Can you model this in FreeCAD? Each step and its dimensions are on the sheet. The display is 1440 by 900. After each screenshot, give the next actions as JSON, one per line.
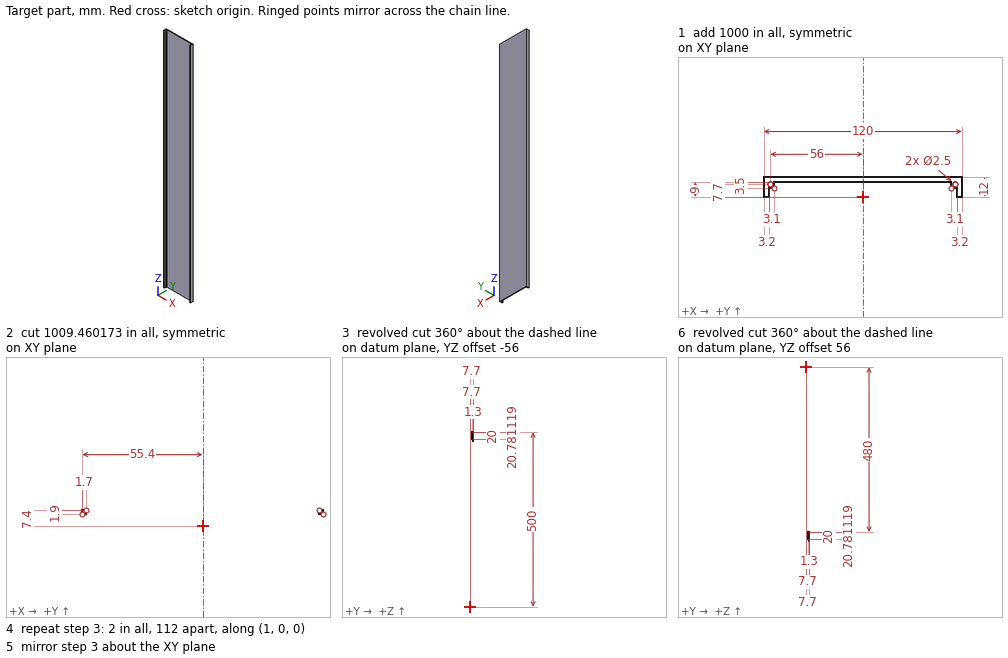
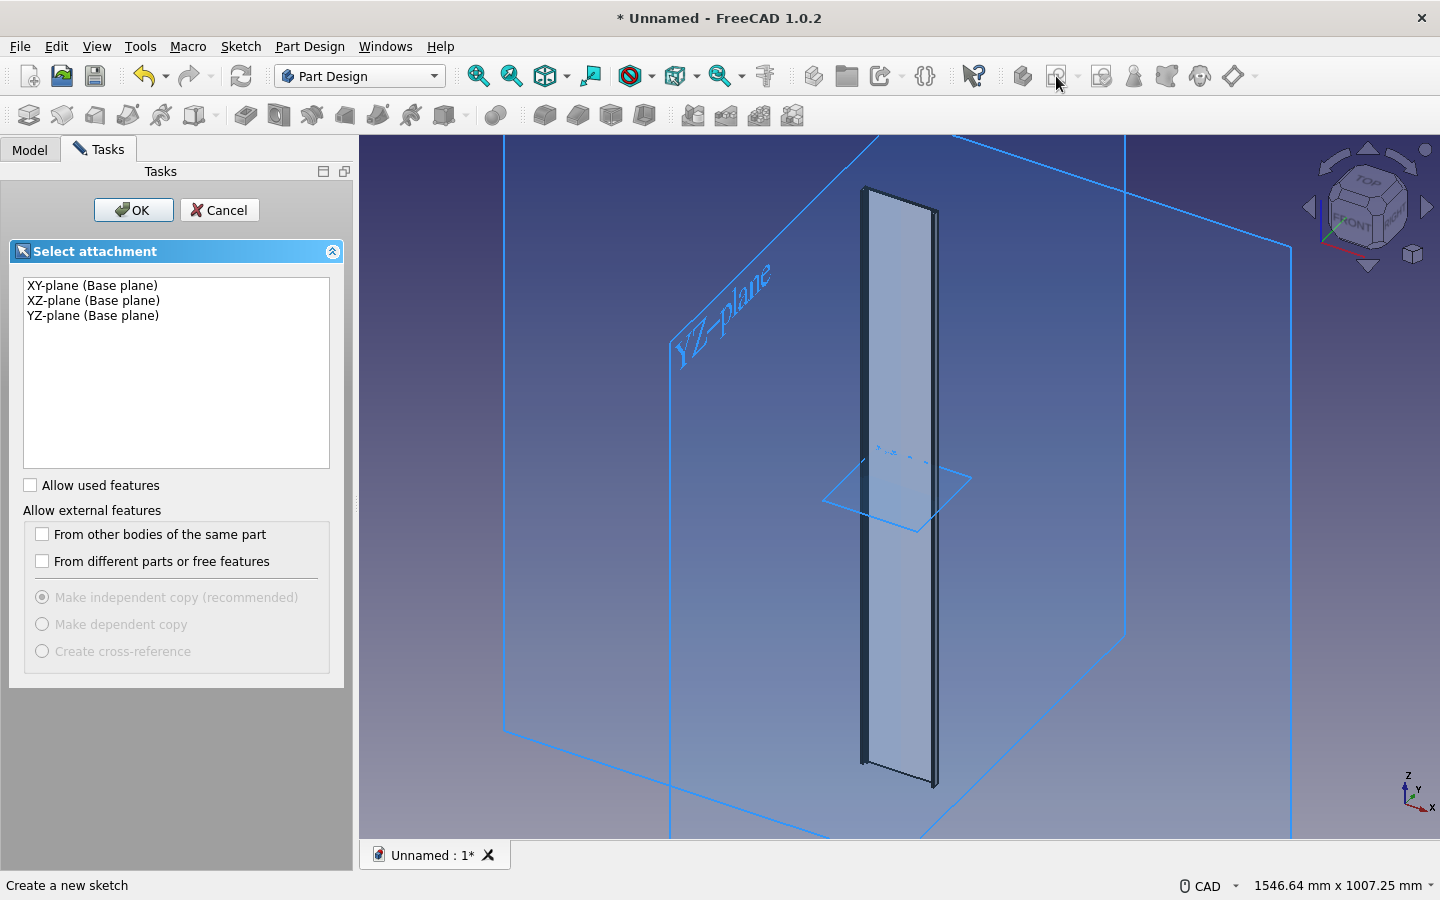
{"action": "left_click", "coordinate": [84, 286]}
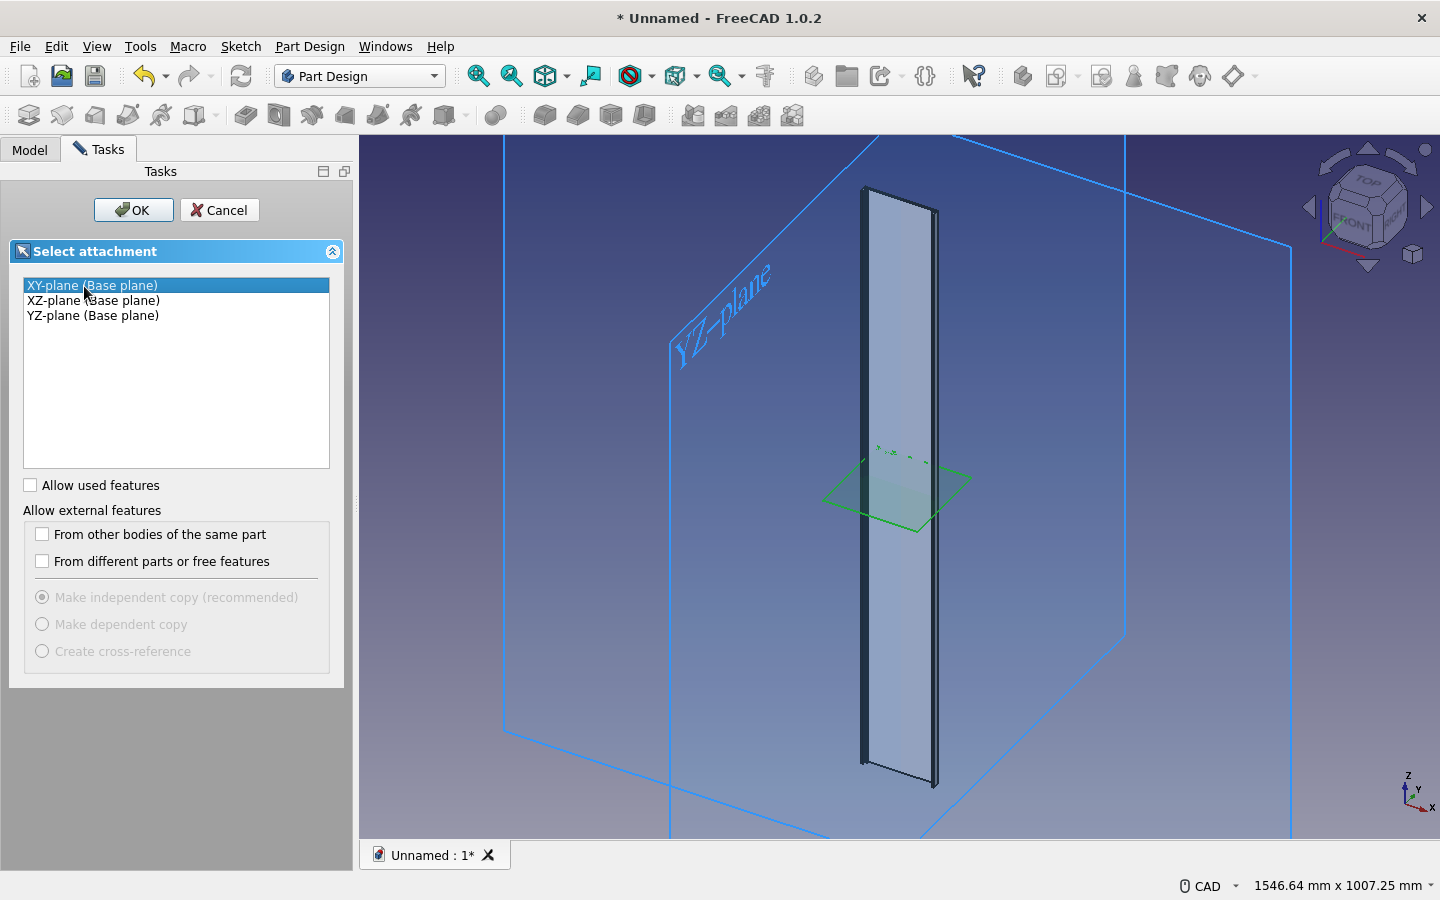
{"action": "left_click", "coordinate": [134, 210]}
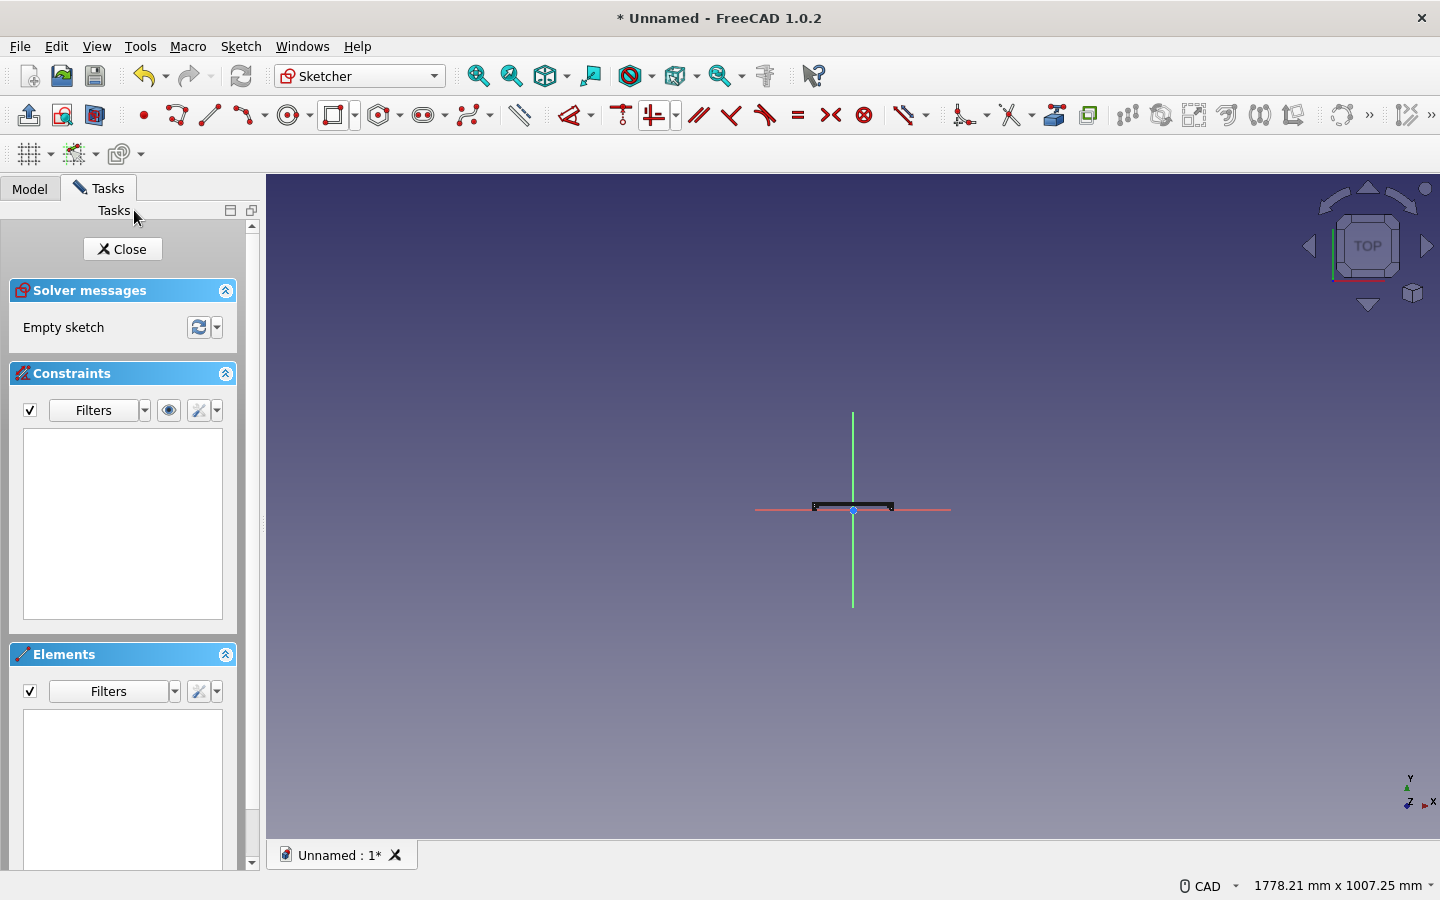
{"action": "left_click", "coordinate": [95, 116]}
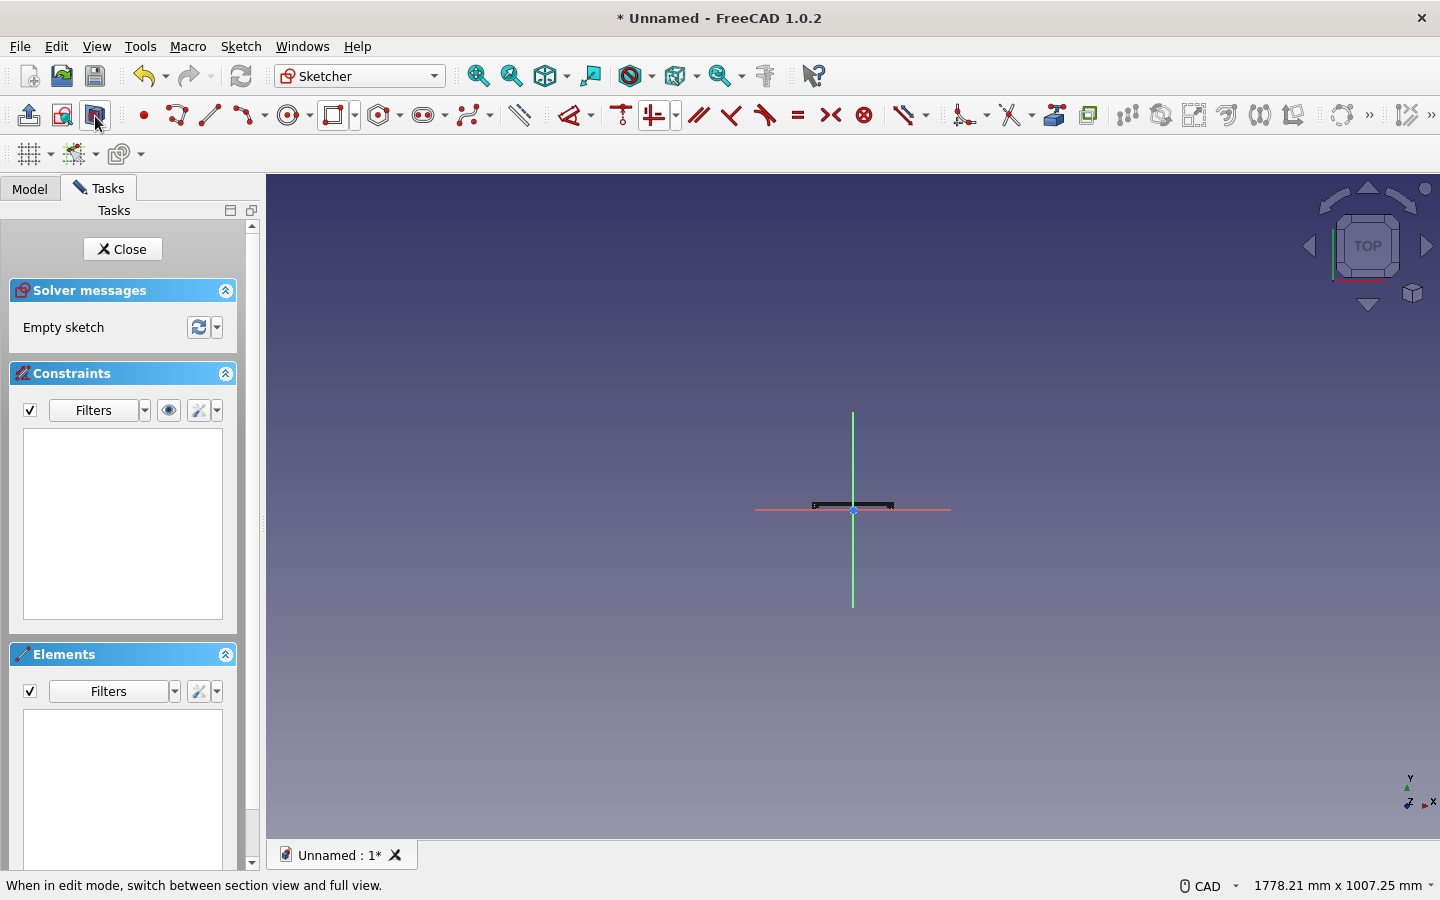
{"action": "scroll", "coordinate": [862, 508], "scroll_direction": "up", "scroll_amount": 11}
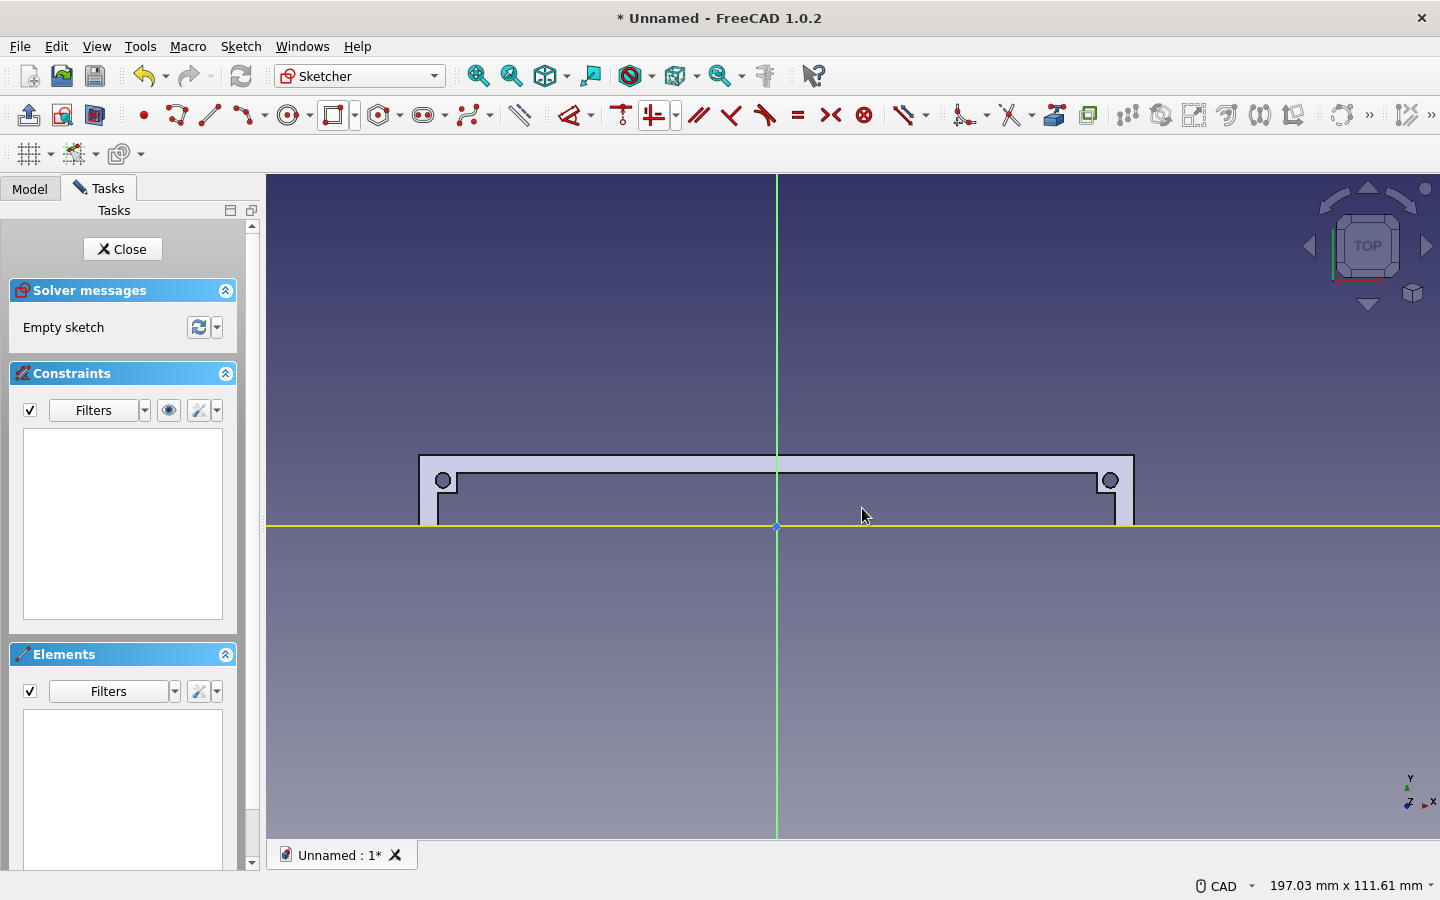
{"action": "left_click", "coordinate": [332, 116]}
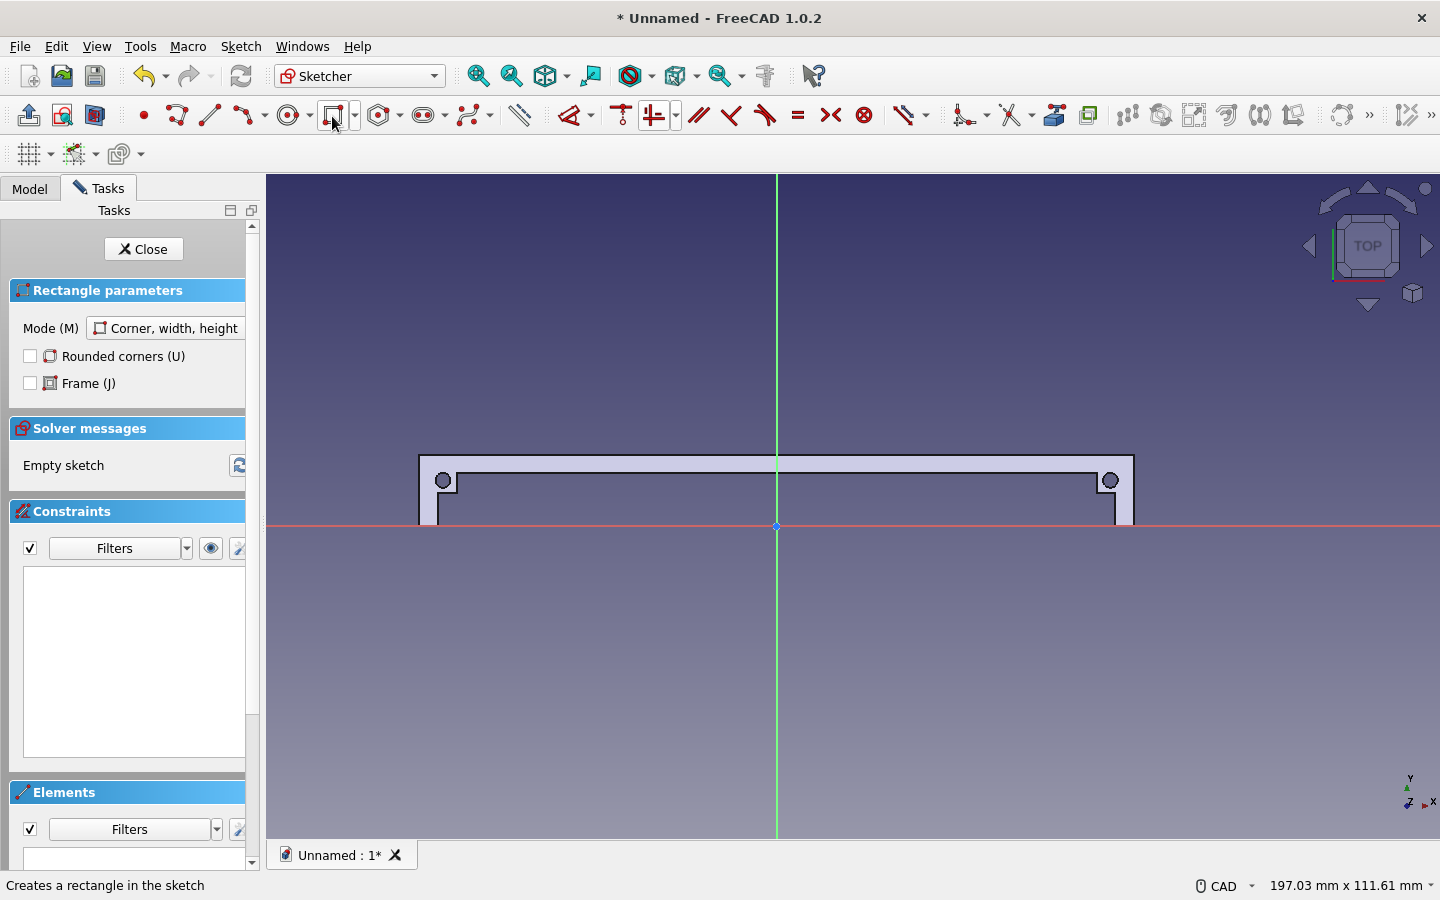
{"action": "scroll", "coordinate": [447, 482], "scroll_direction": "up", "scroll_amount": 3}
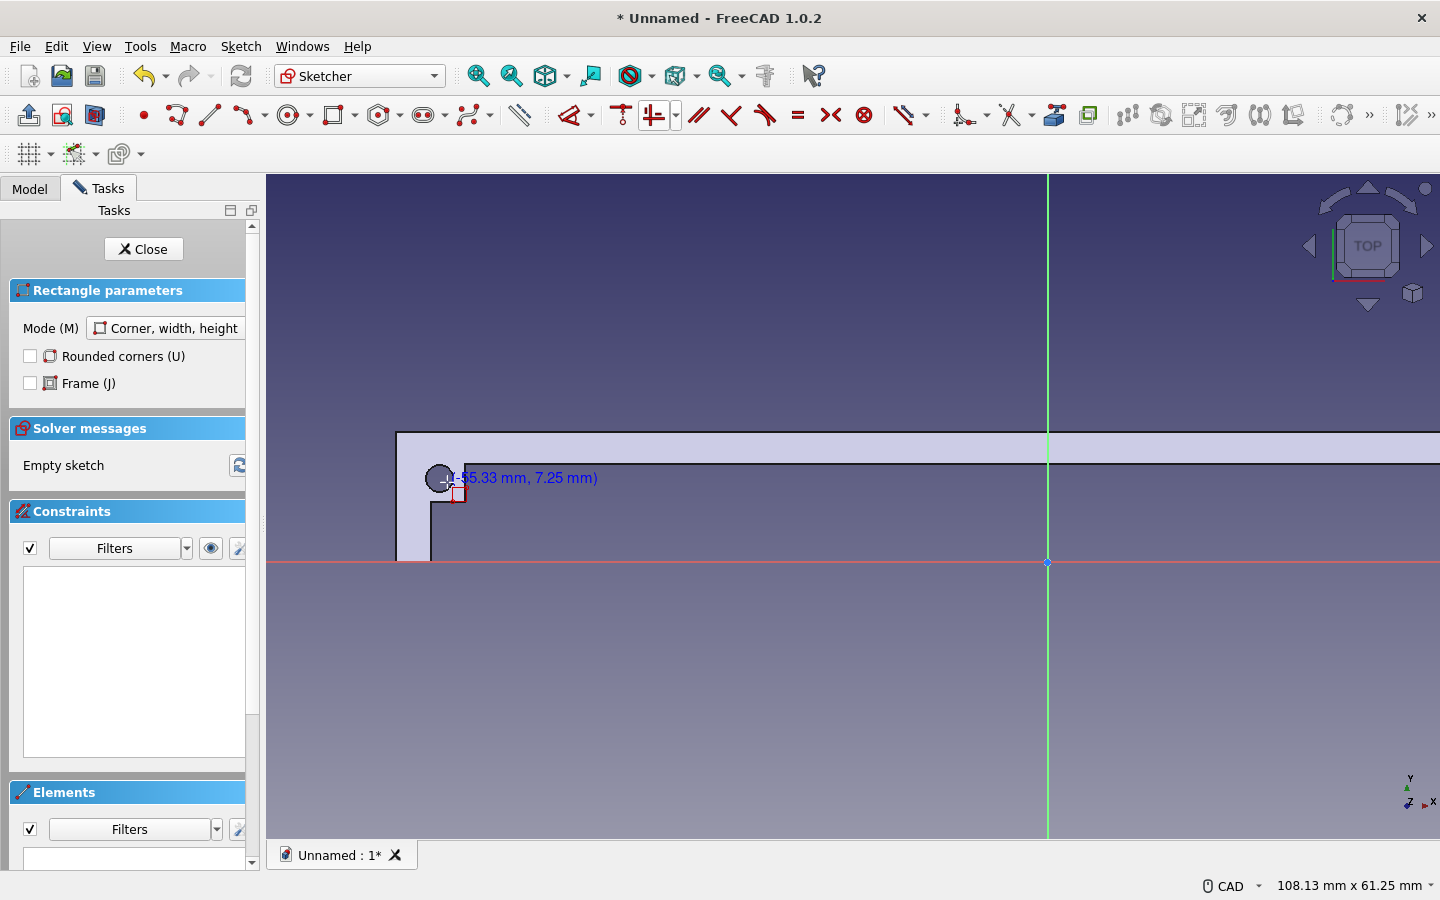
{"action": "left_click", "coordinate": [446, 482]}
{"action": "left_click", "coordinate": [465, 502]}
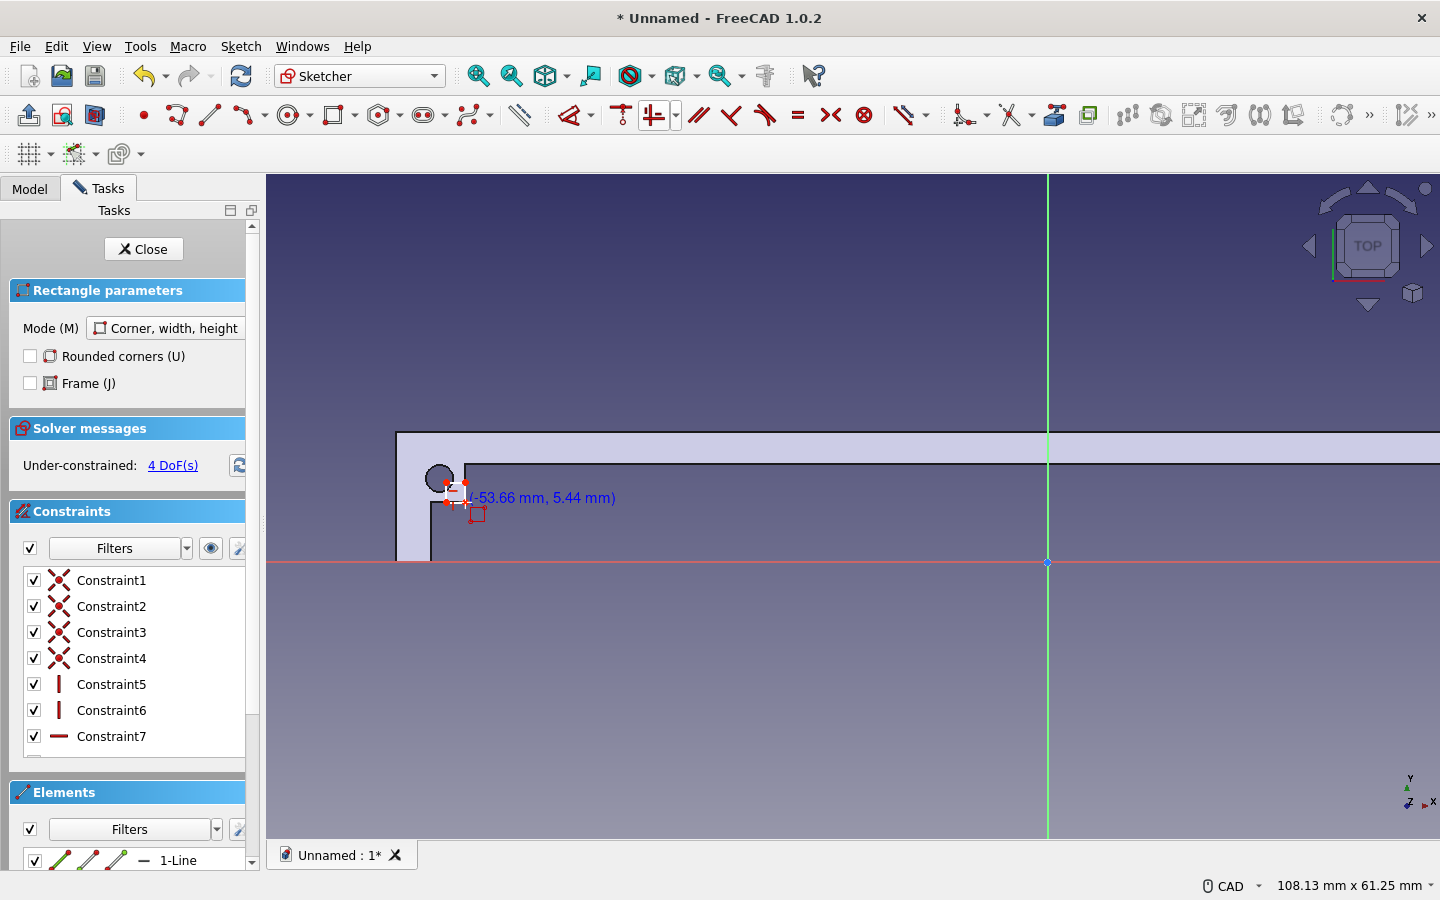
{"action": "scroll", "coordinate": [464, 488], "scroll_direction": "down", "scroll_amount": 3}